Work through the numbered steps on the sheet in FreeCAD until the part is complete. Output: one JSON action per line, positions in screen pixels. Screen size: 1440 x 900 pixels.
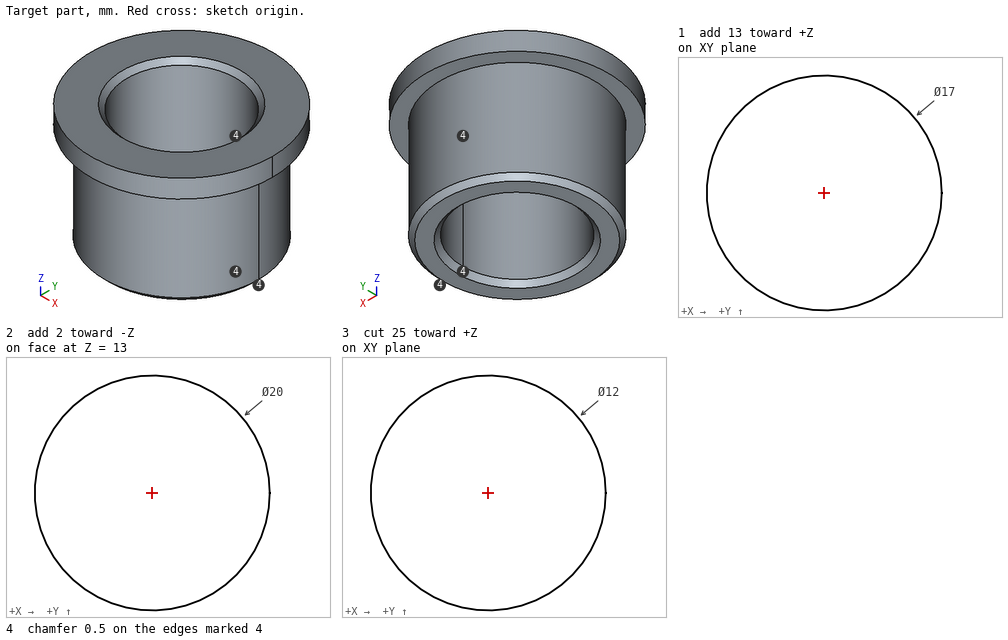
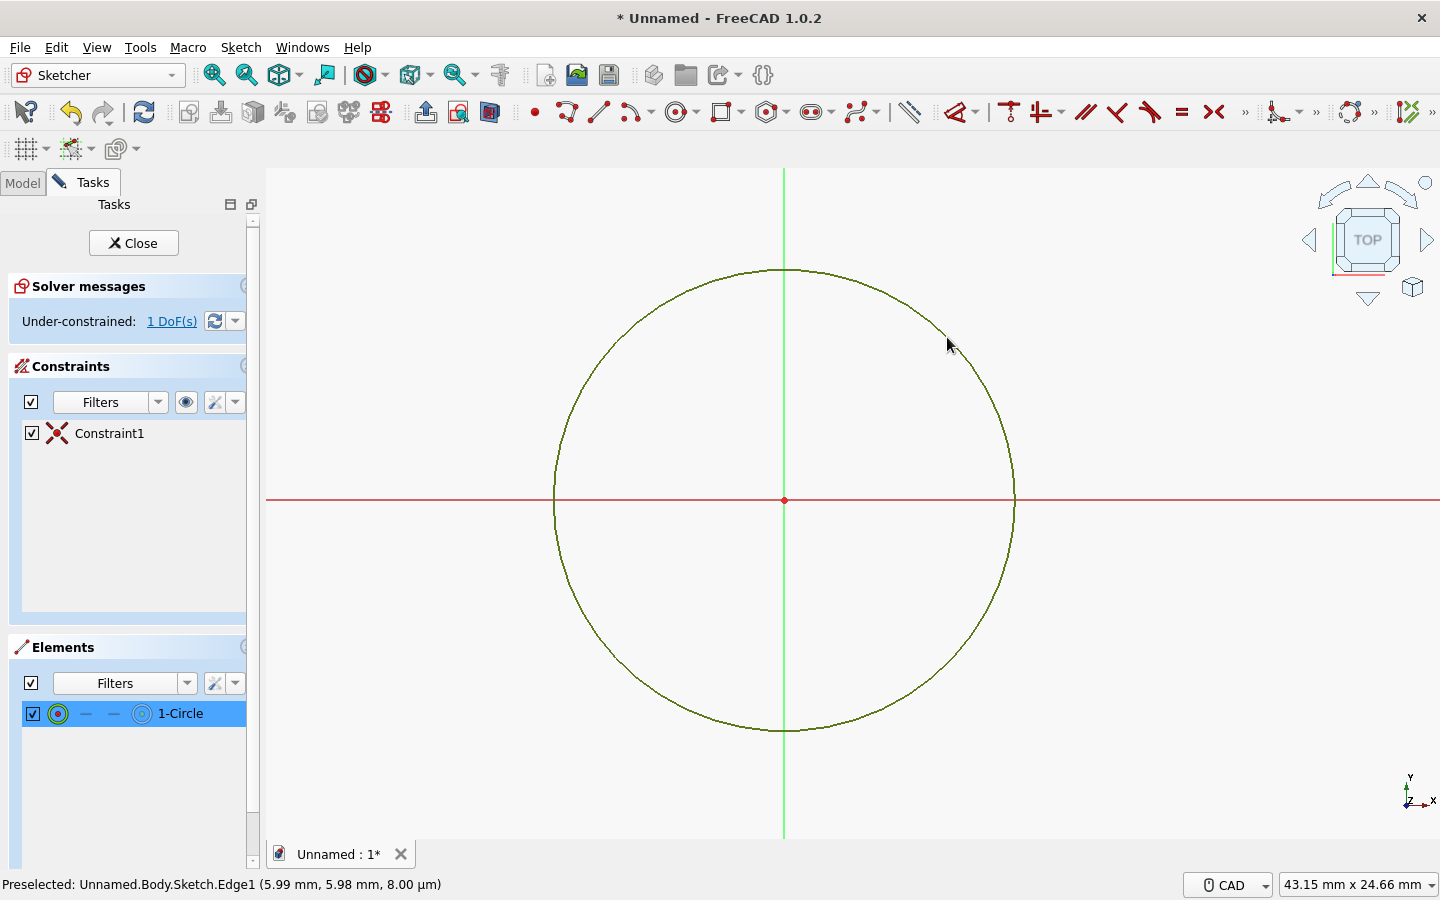
{"action": "key", "text": "k o"}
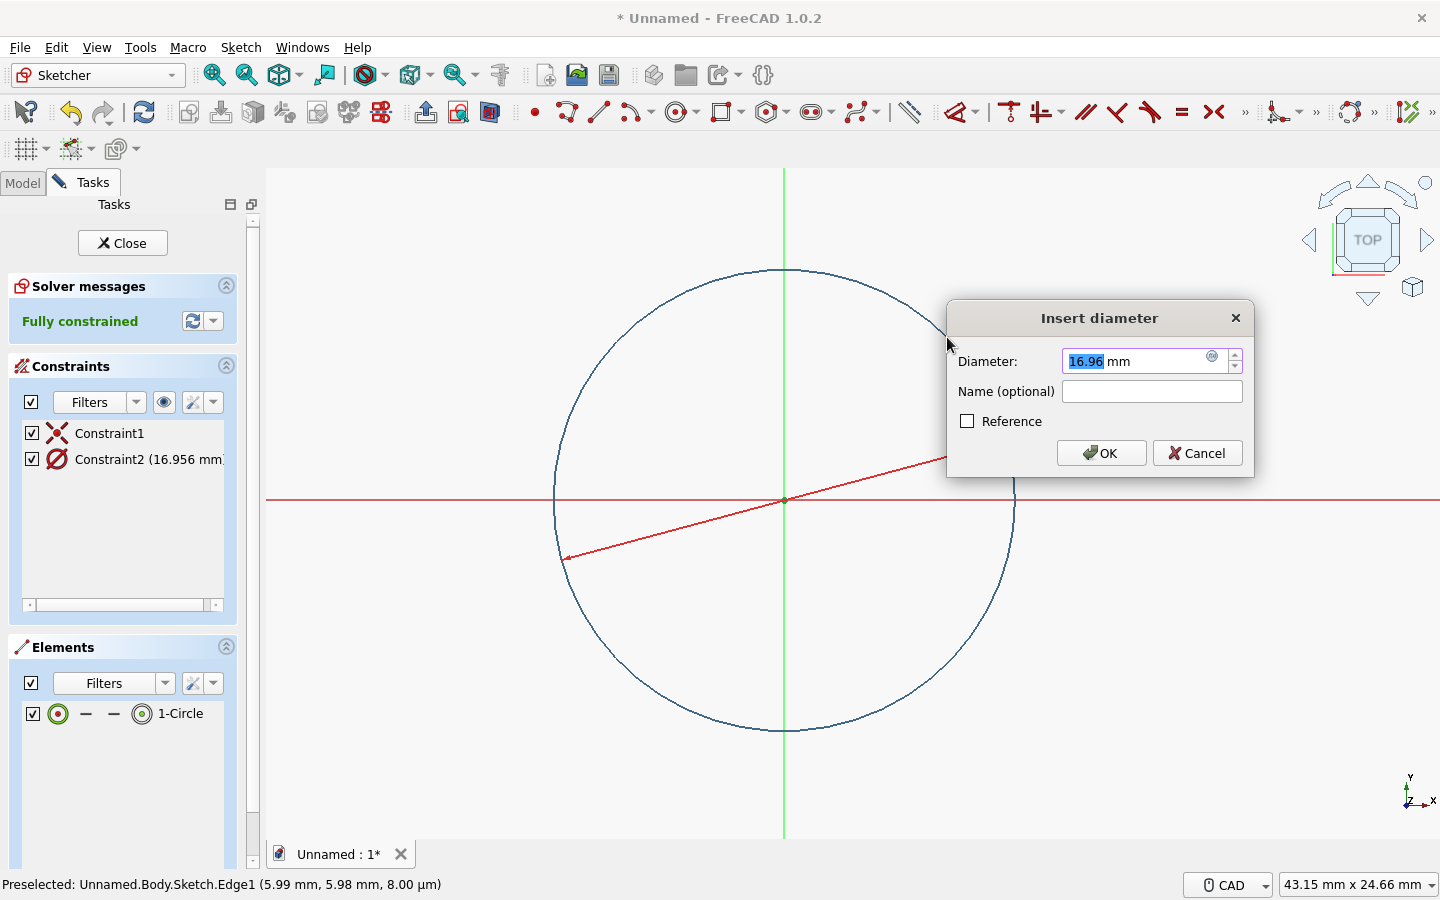
{"action": "type", "text": "17"}
{"action": "key", "text": "Return"}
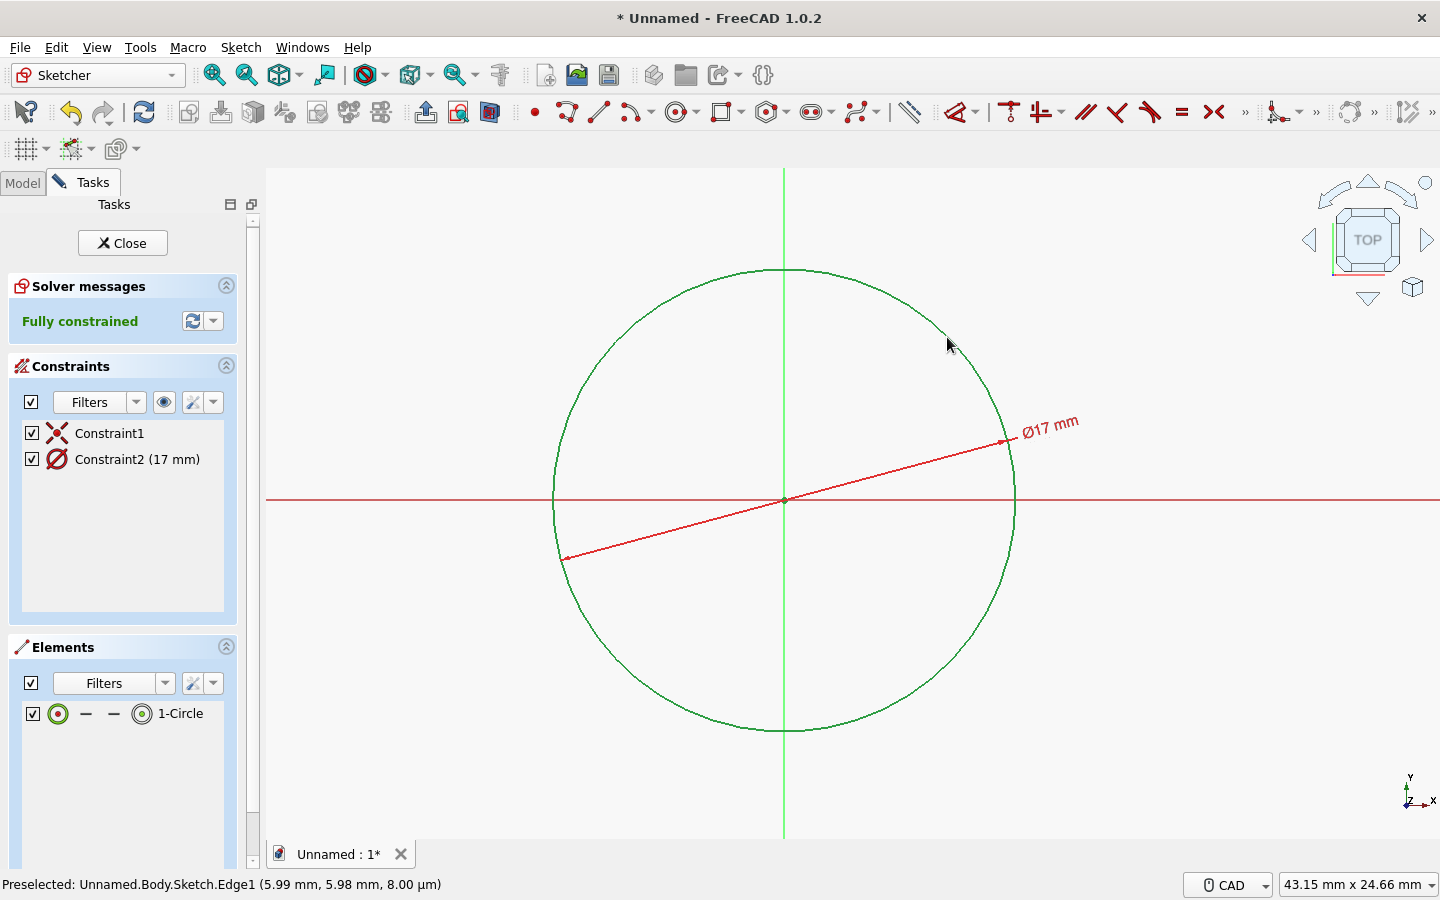
{"action": "left_click", "coordinate": [123, 243]}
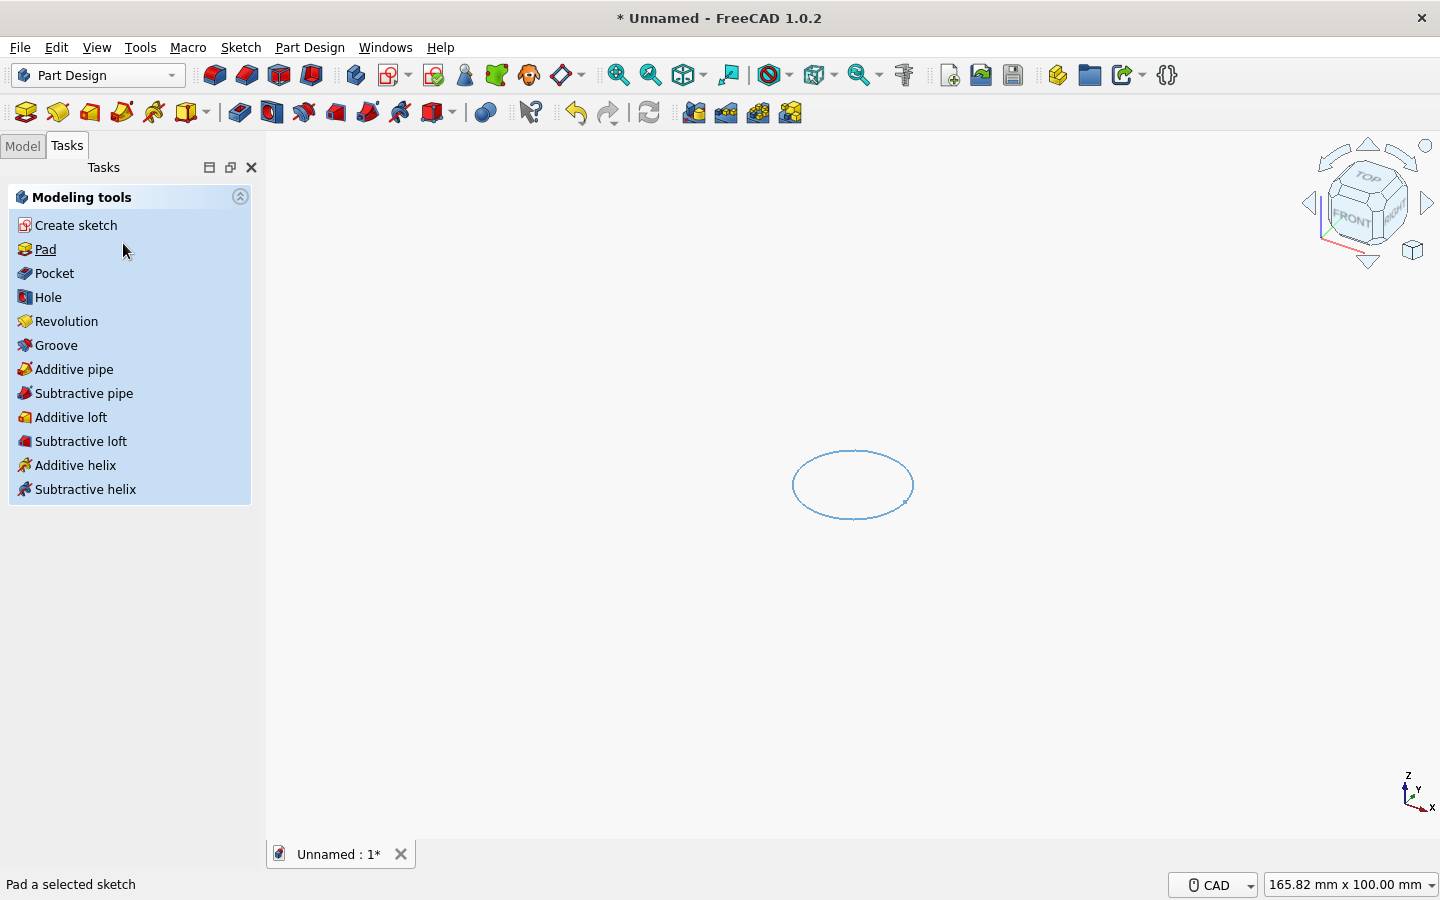
{"action": "left_click", "coordinate": [26, 112]}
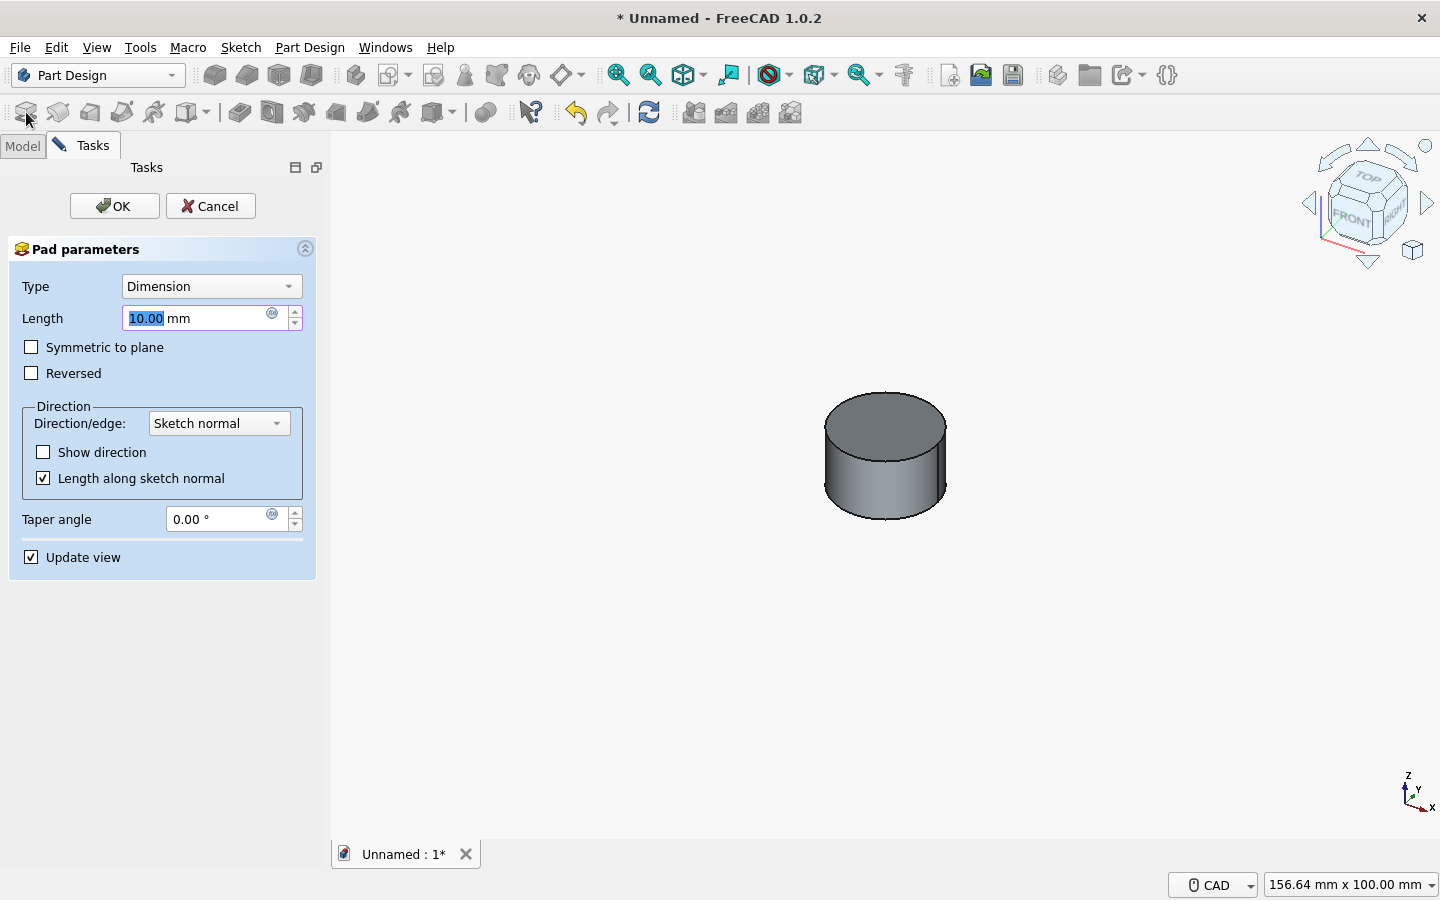
{"action": "type", "text": "13"}
{"action": "key", "text": "Tab"}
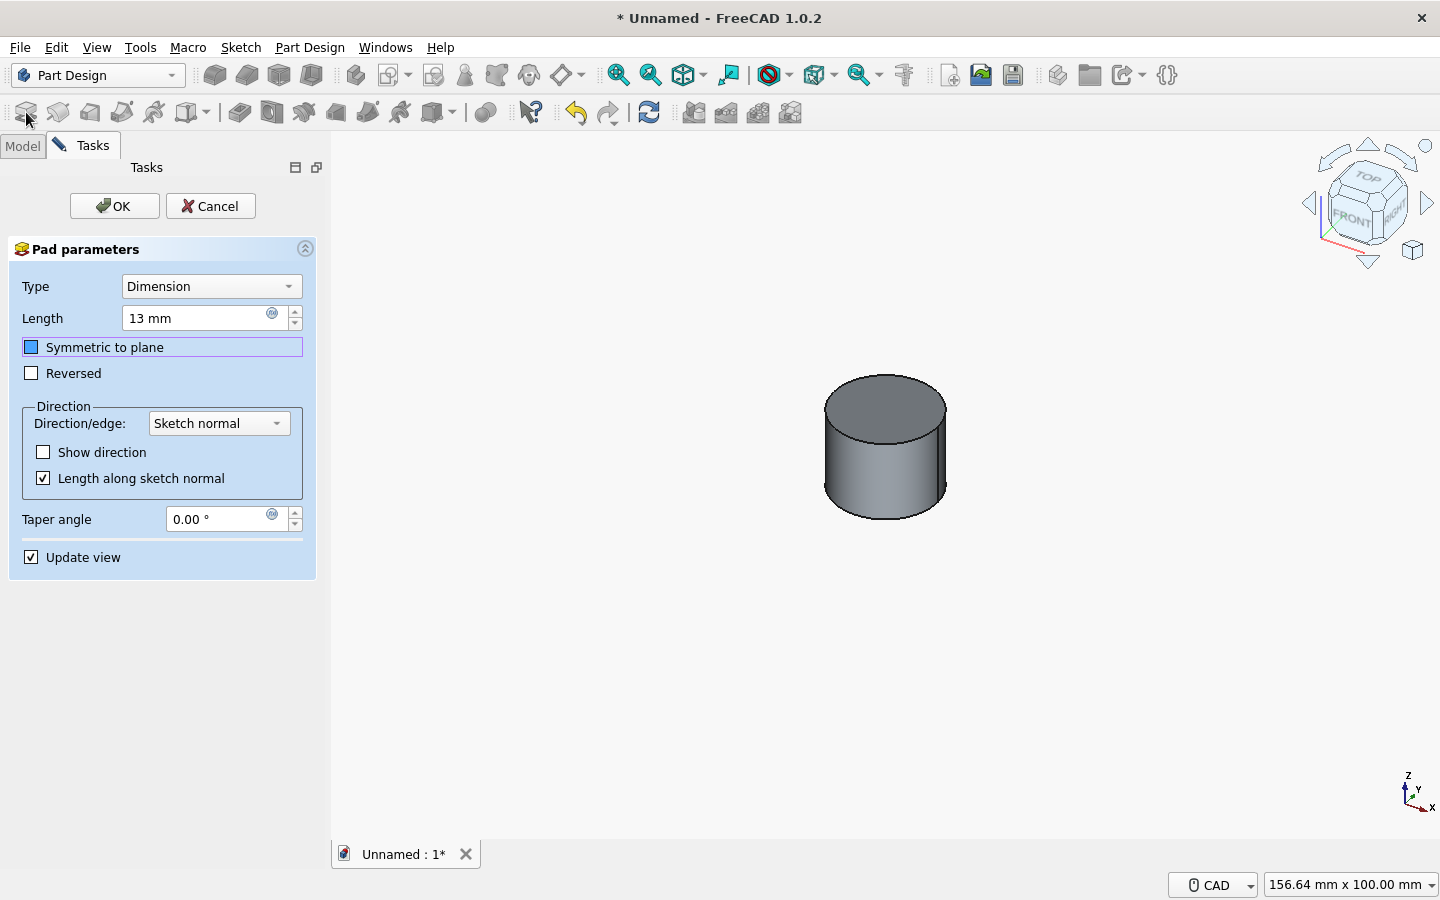
{"action": "left_click", "coordinate": [115, 206]}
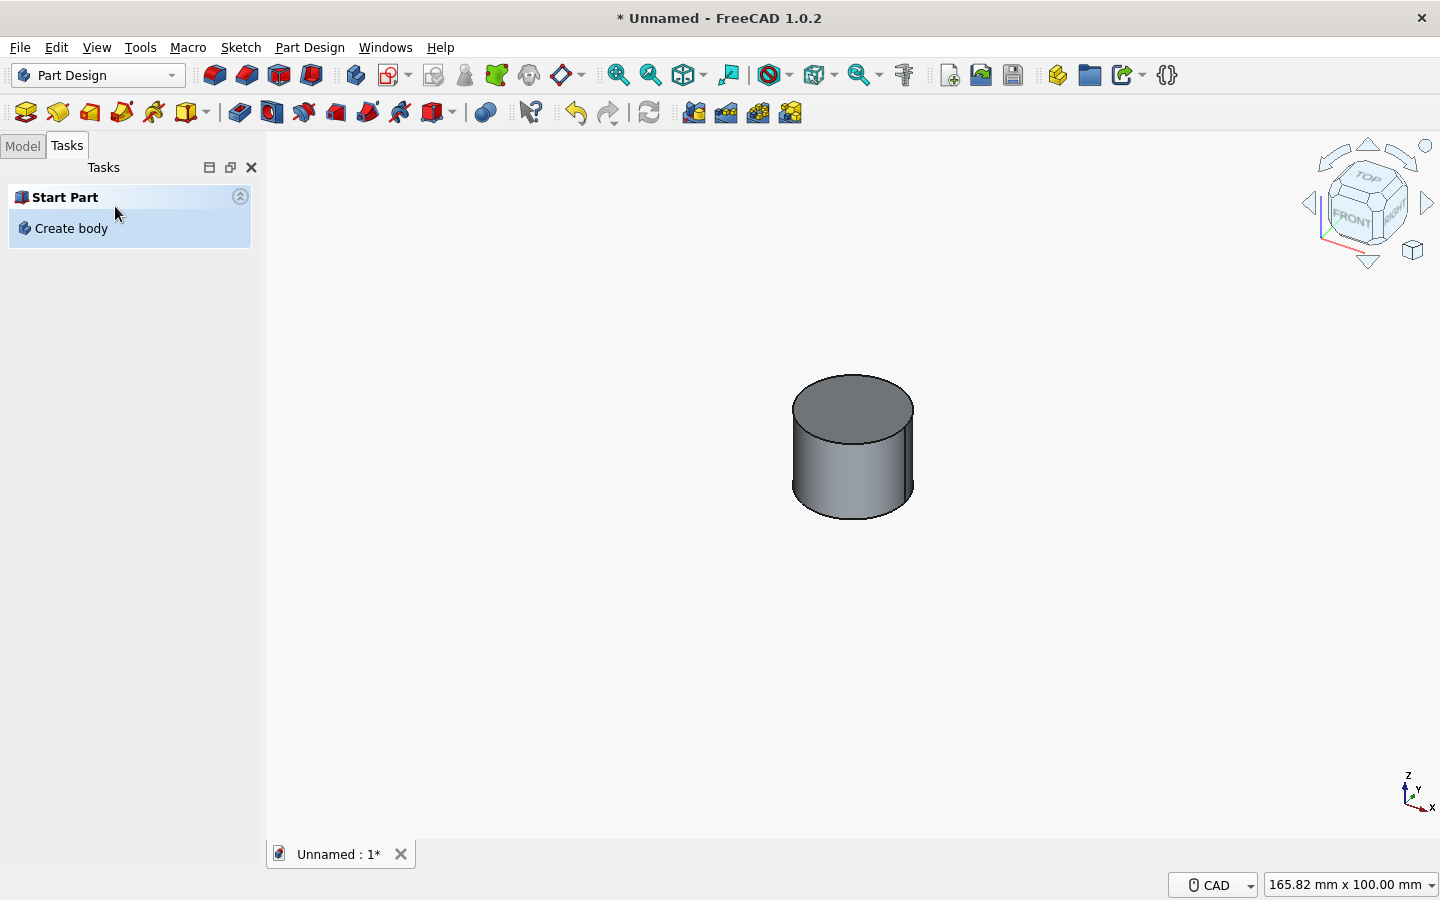
{"action": "key", "text": "v f"}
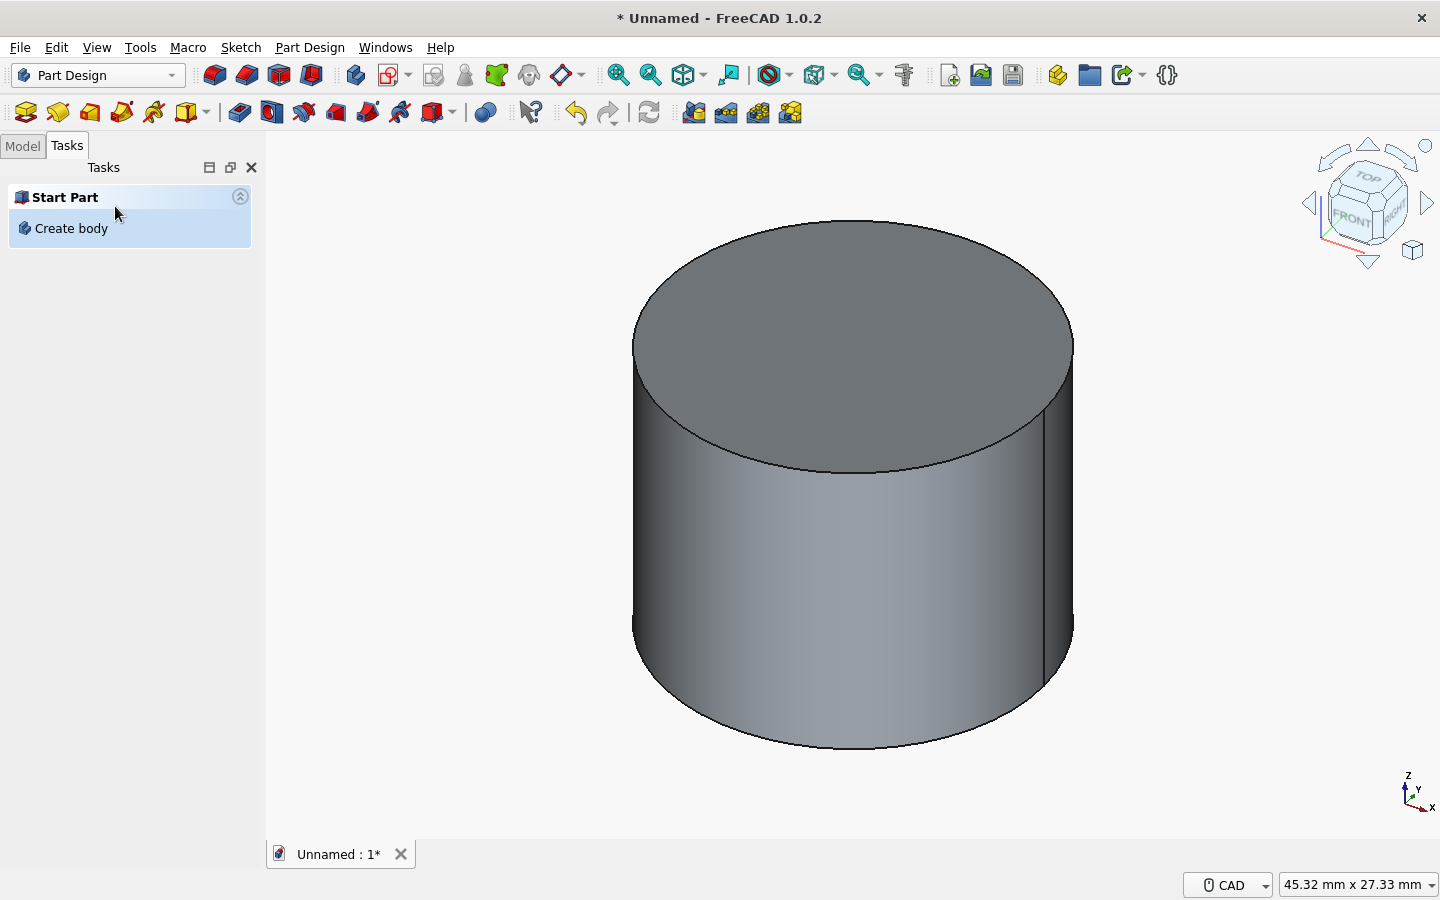
{"action": "left_click", "coordinate": [853, 346]}